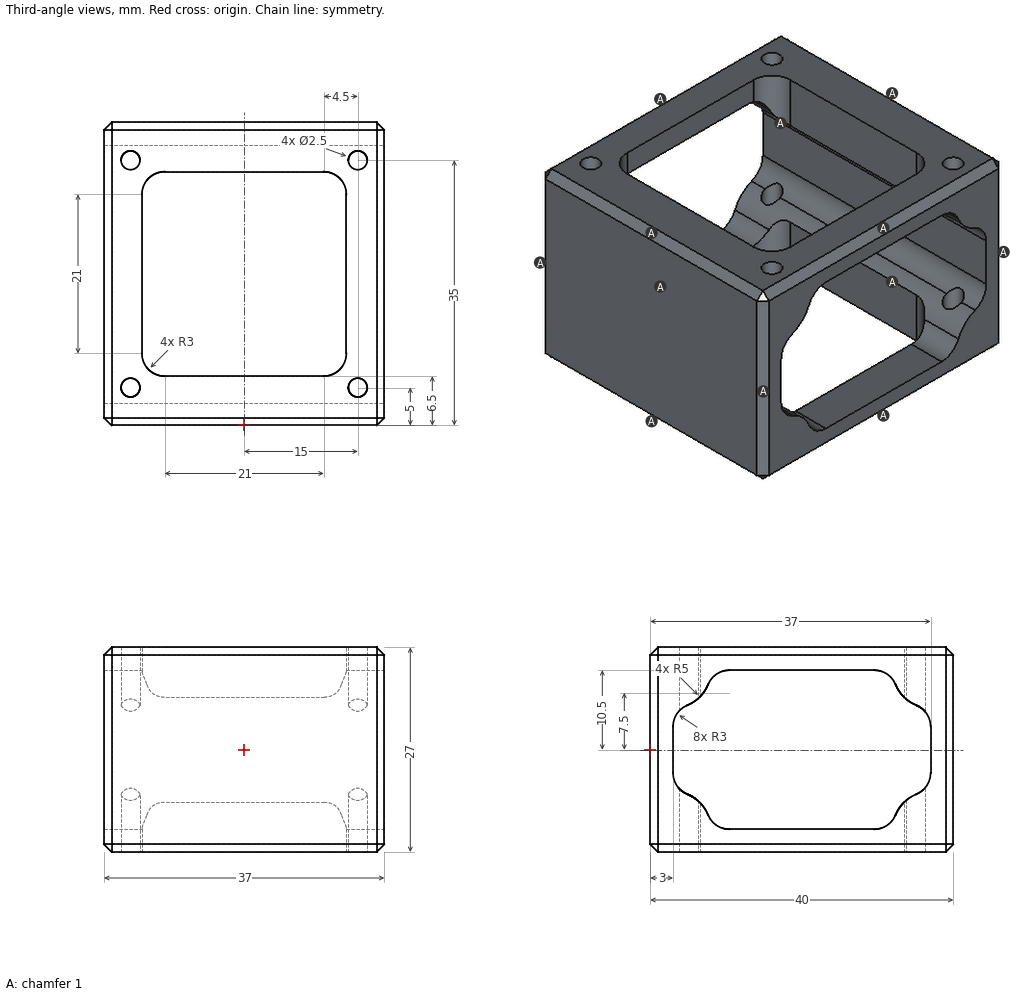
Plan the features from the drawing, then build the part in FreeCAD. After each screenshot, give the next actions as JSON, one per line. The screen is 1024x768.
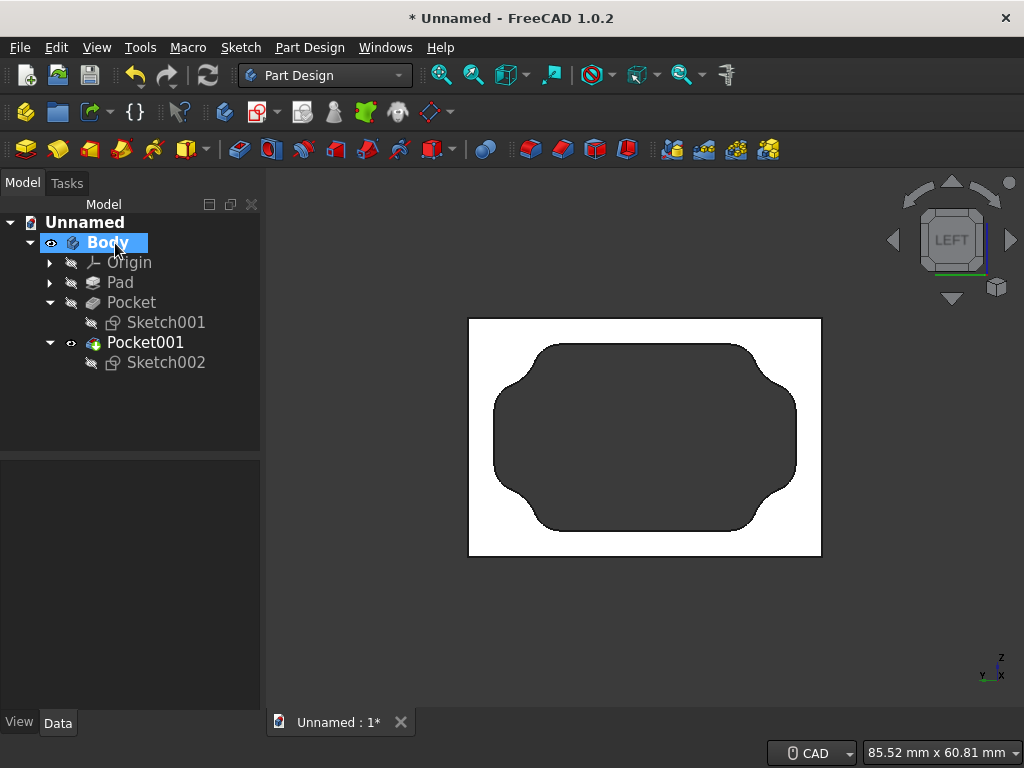
{"action": "left_click", "coordinate": [645, 317]}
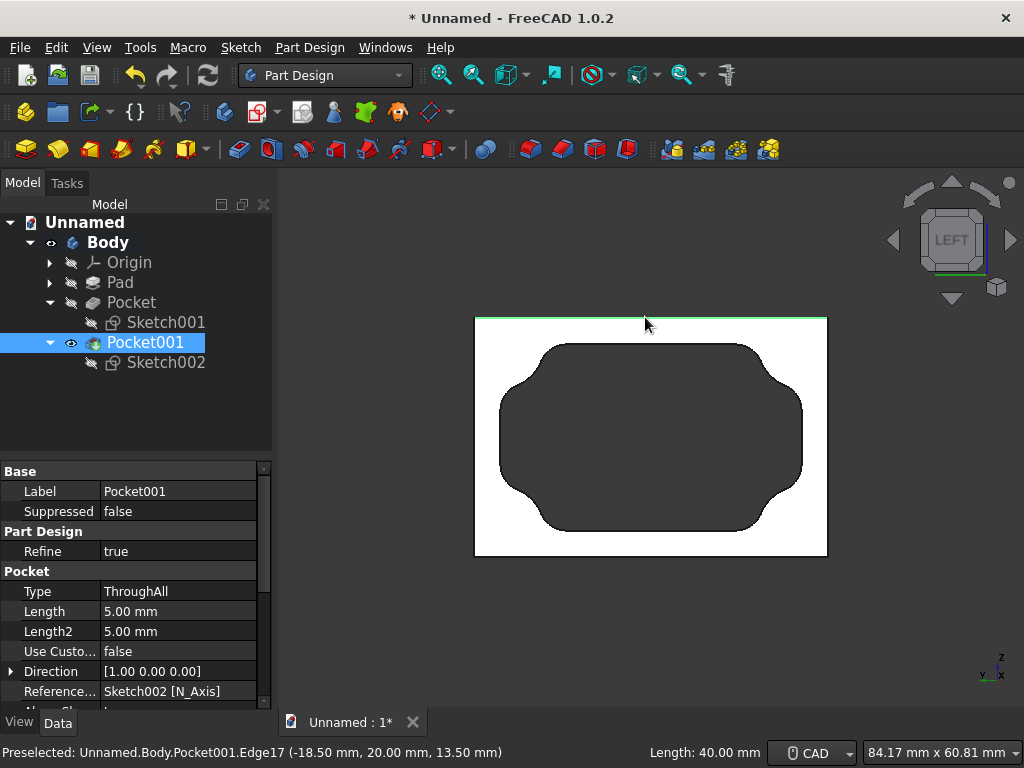
{"action": "left_click", "coordinate": [651, 556], "text": "ctrl"}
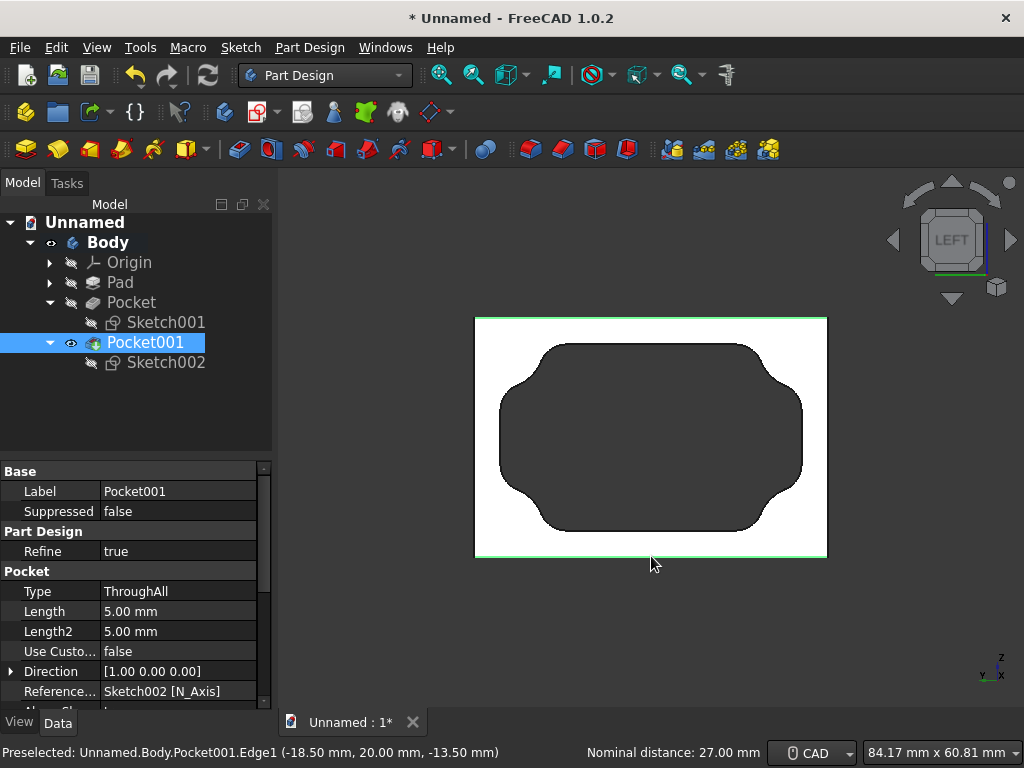
{"action": "key", "text": "0"}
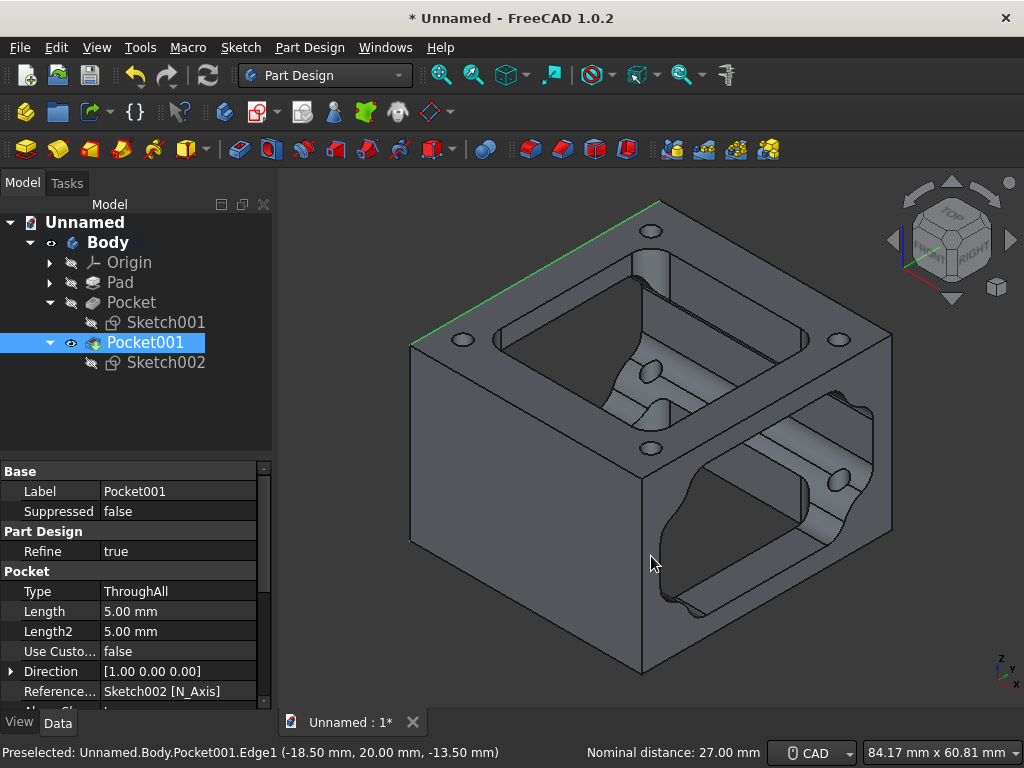
{"action": "left_click", "coordinate": [526, 509], "text": "ctrl"}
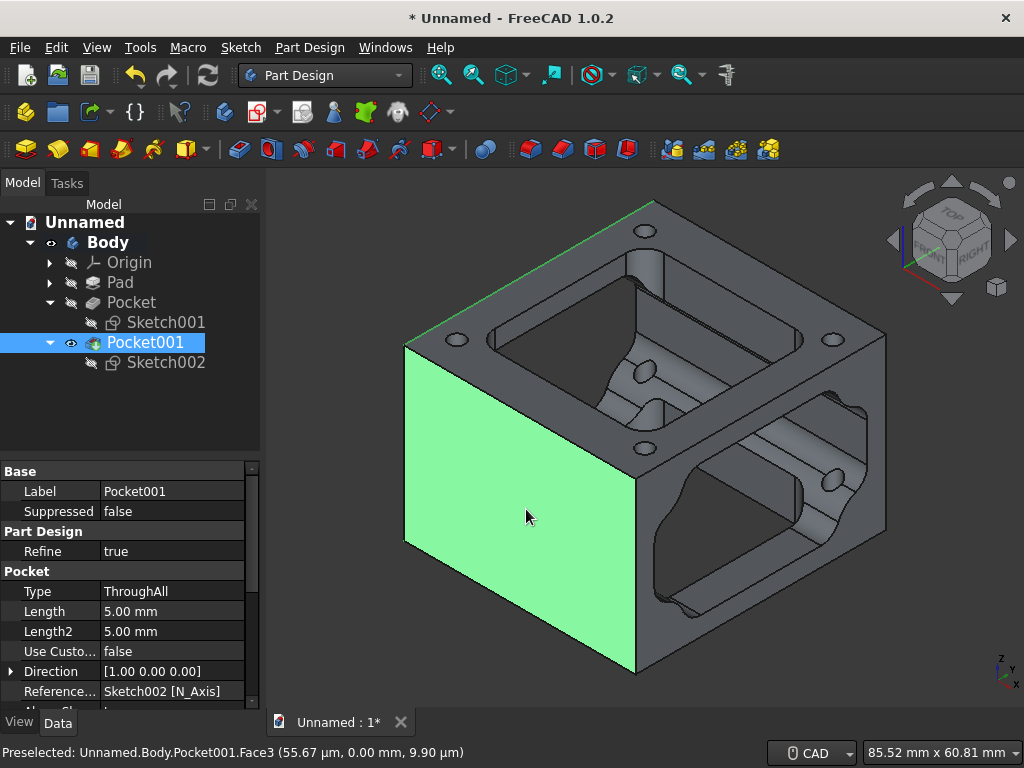
{"action": "left_click", "coordinate": [761, 406], "text": "ctrl"}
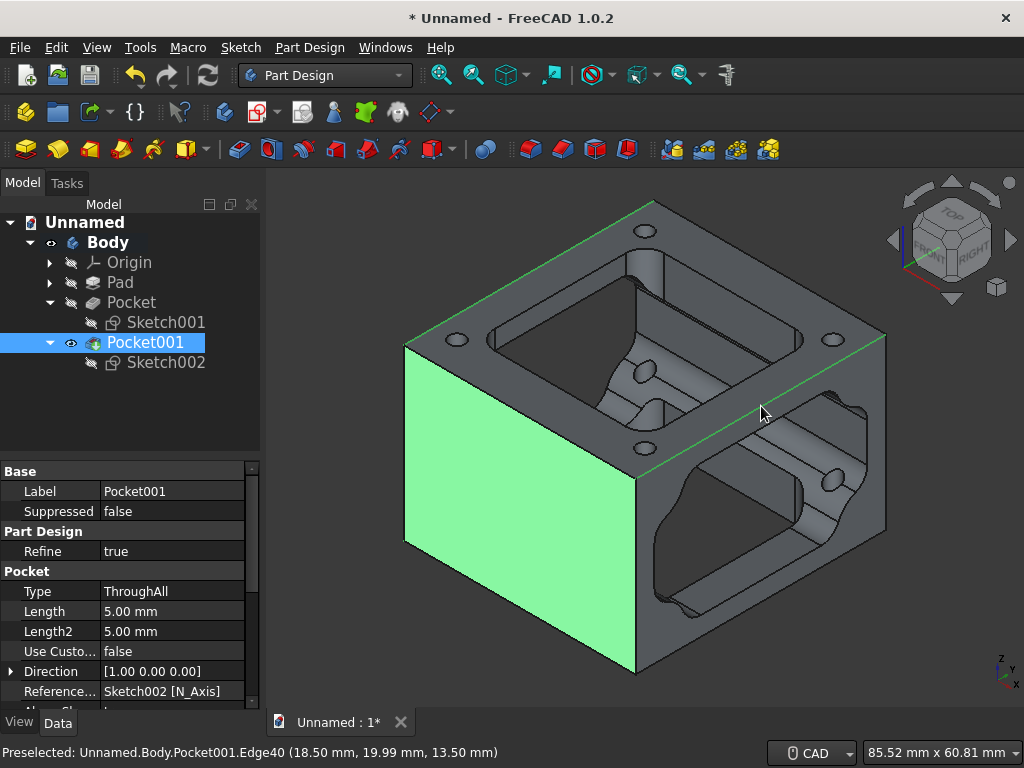
{"action": "key", "text": "2"}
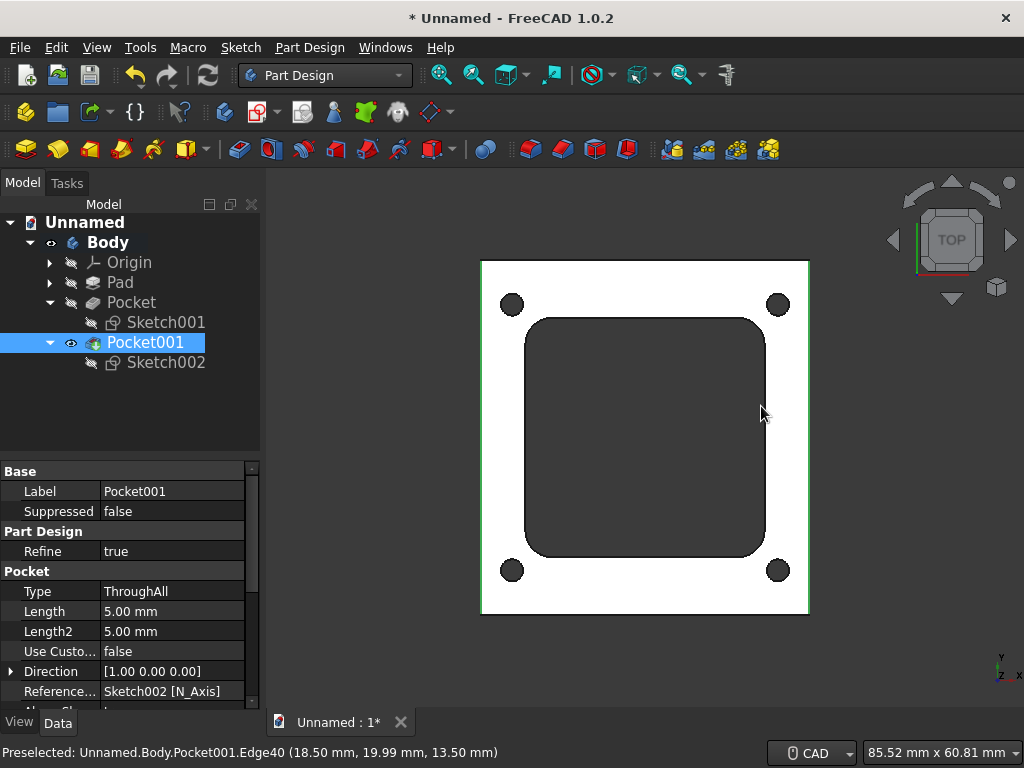
{"action": "key", "text": "1"}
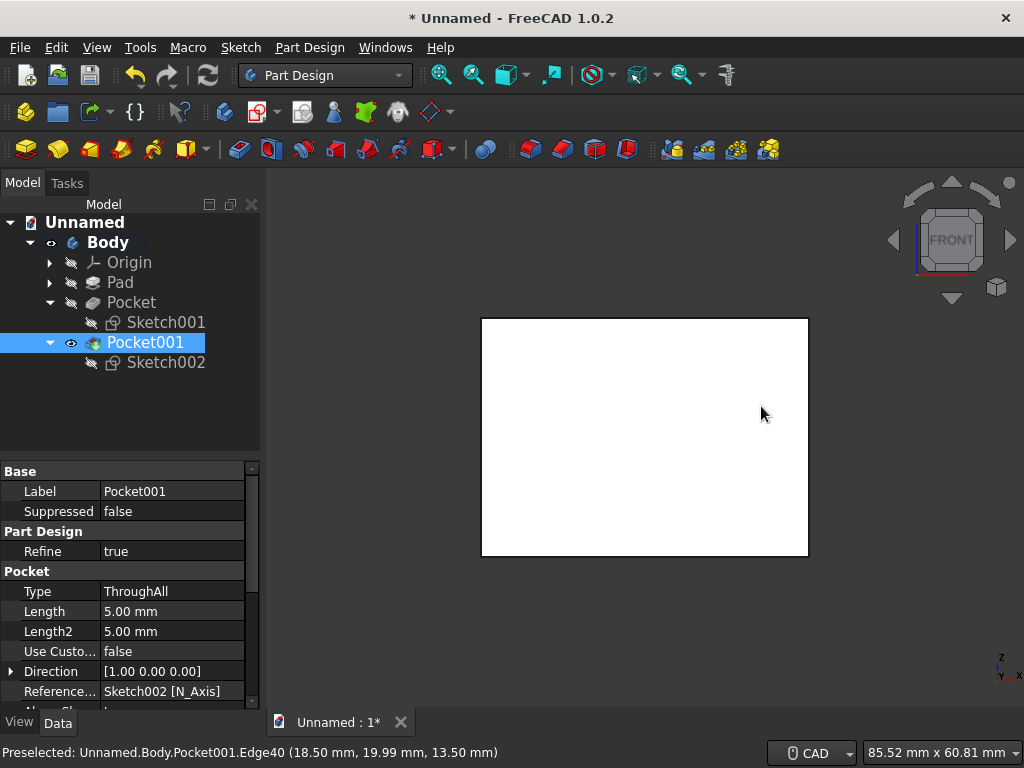
{"action": "left_click", "coordinate": [442, 76]}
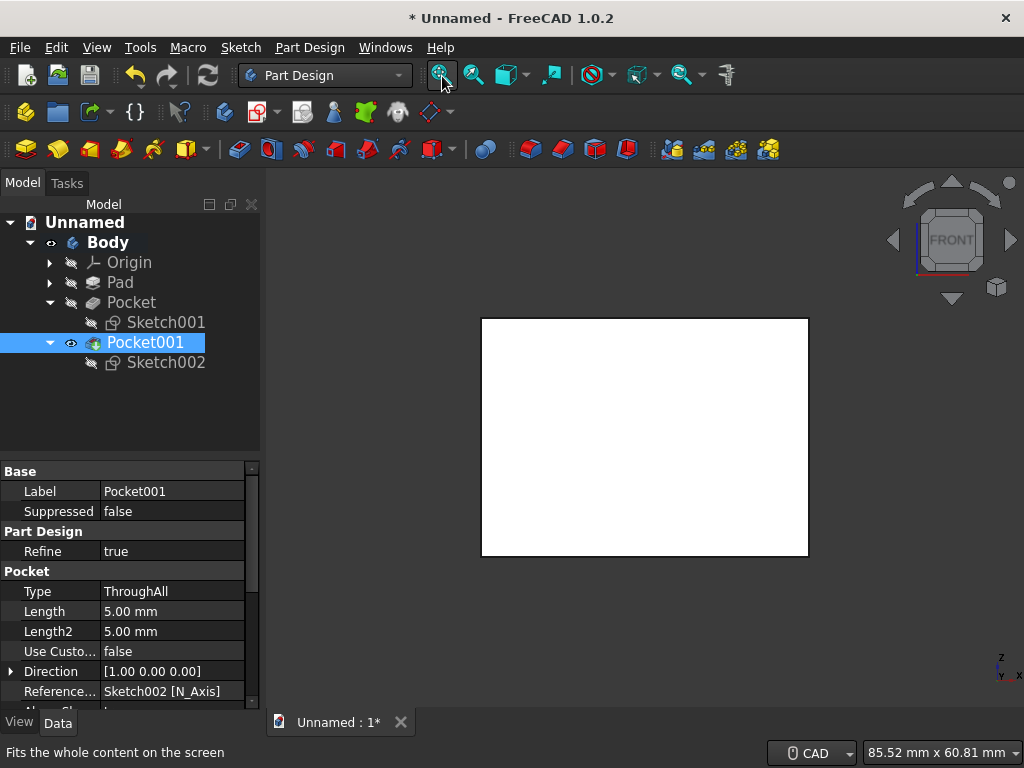
{"action": "key", "text": "3"}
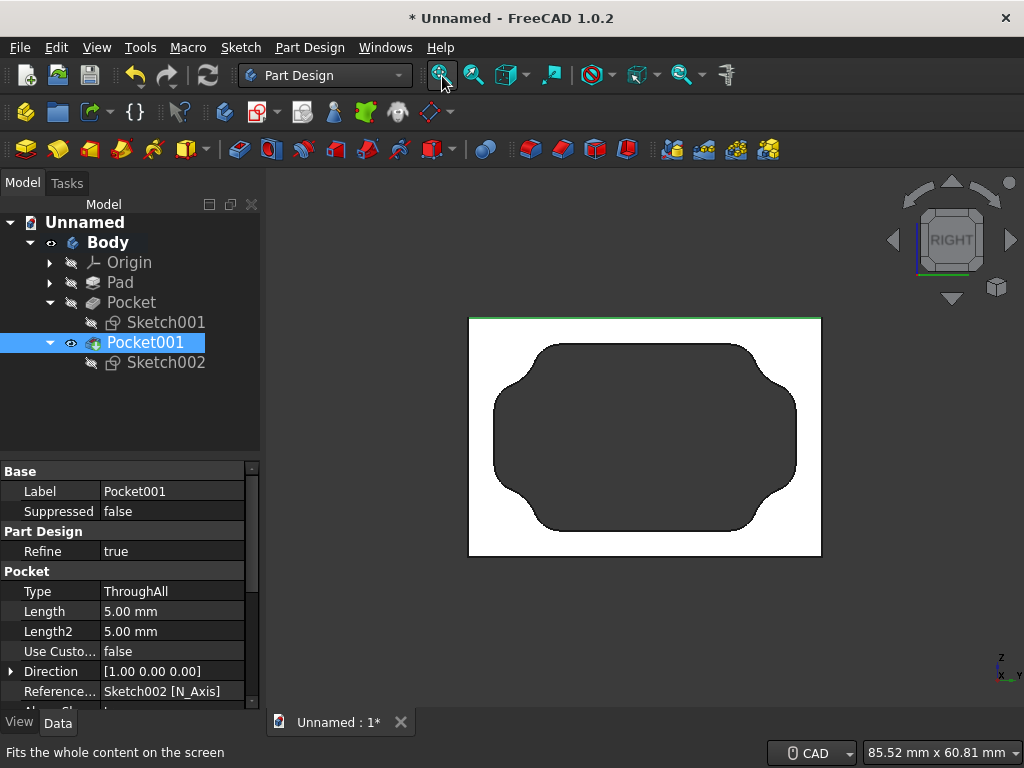
{"action": "left_click", "coordinate": [645, 556], "text": "ctrl"}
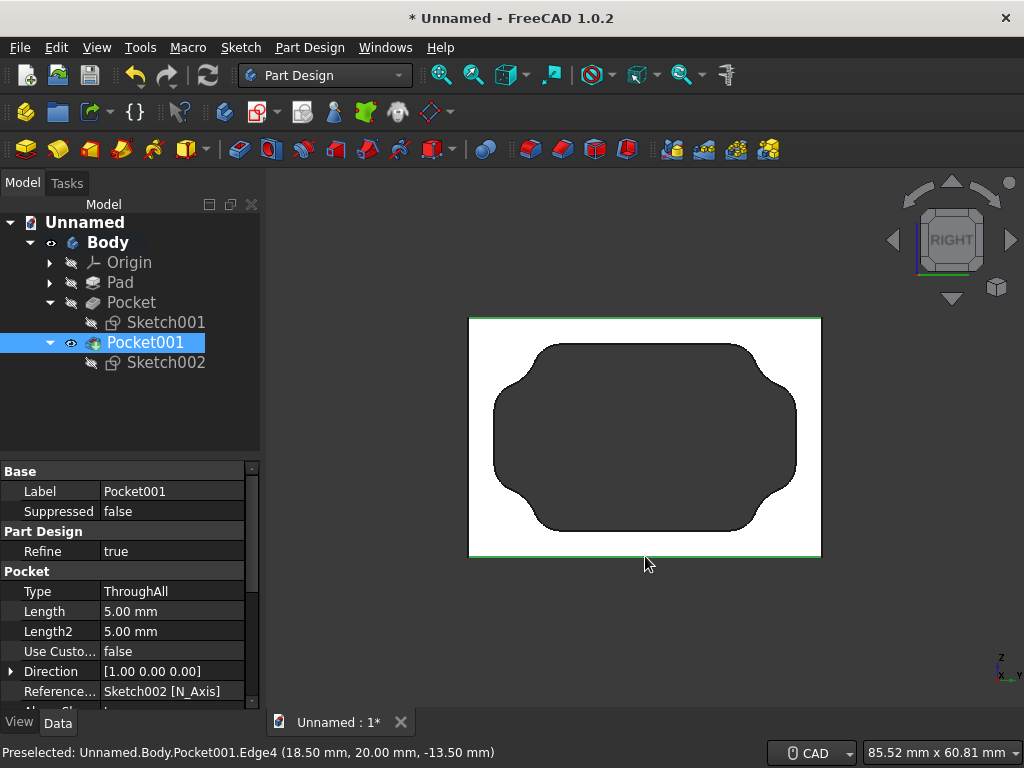
{"action": "key", "text": "5"}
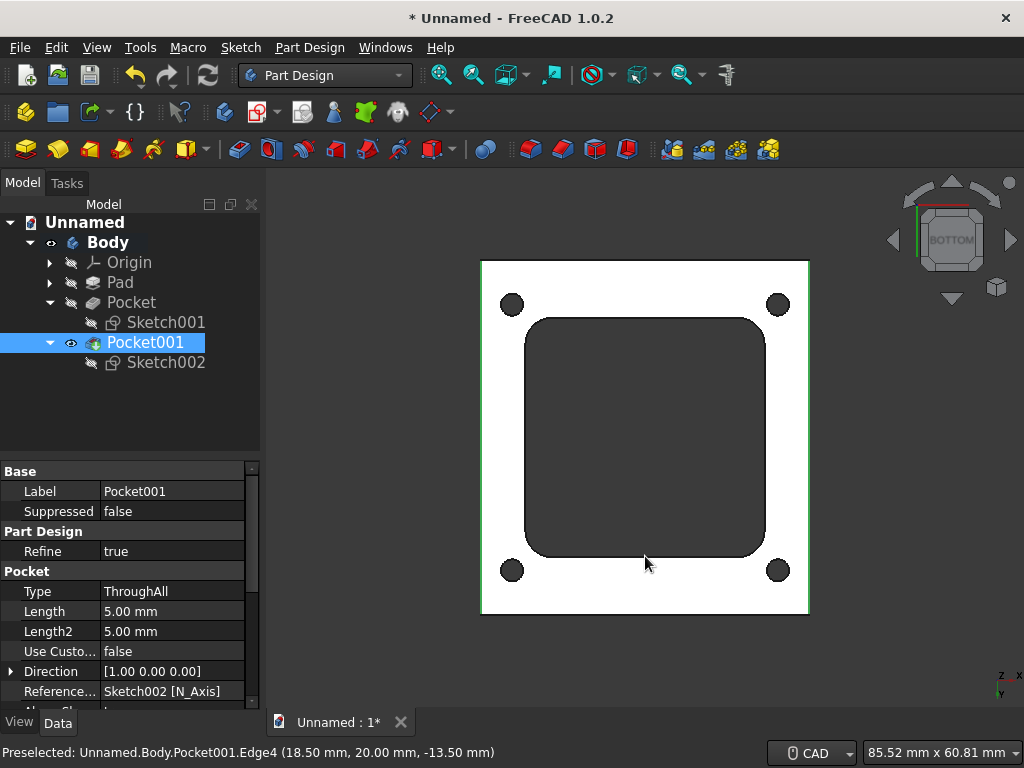
{"action": "key", "text": "4"}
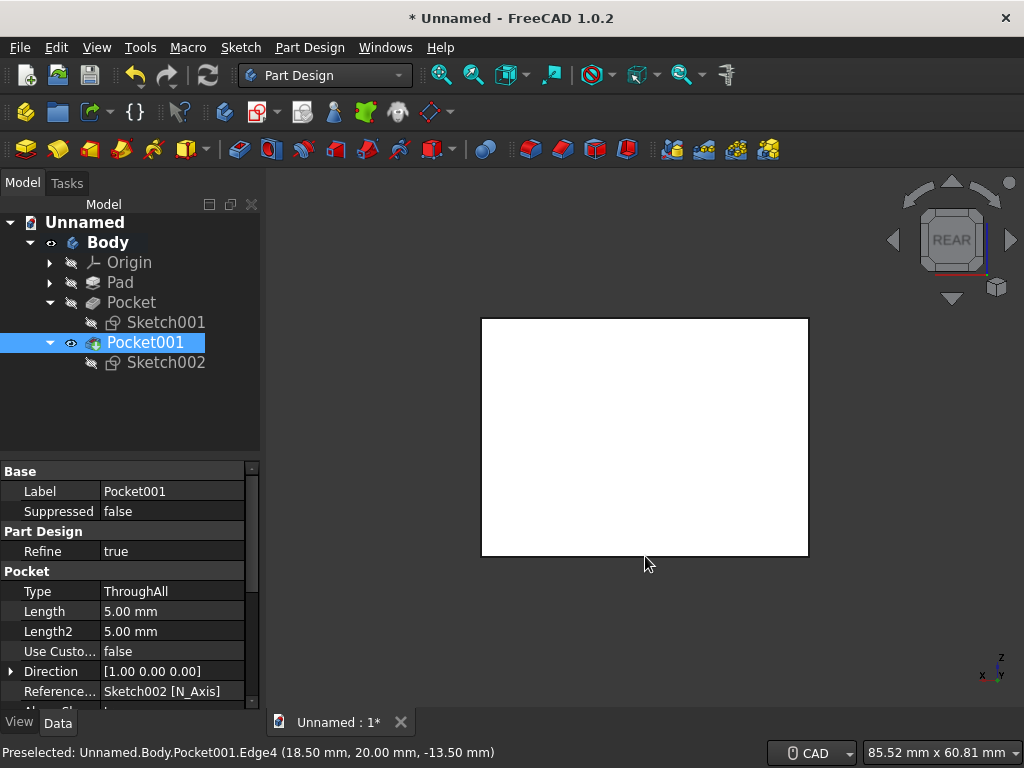
{"action": "key", "text": "v f"}